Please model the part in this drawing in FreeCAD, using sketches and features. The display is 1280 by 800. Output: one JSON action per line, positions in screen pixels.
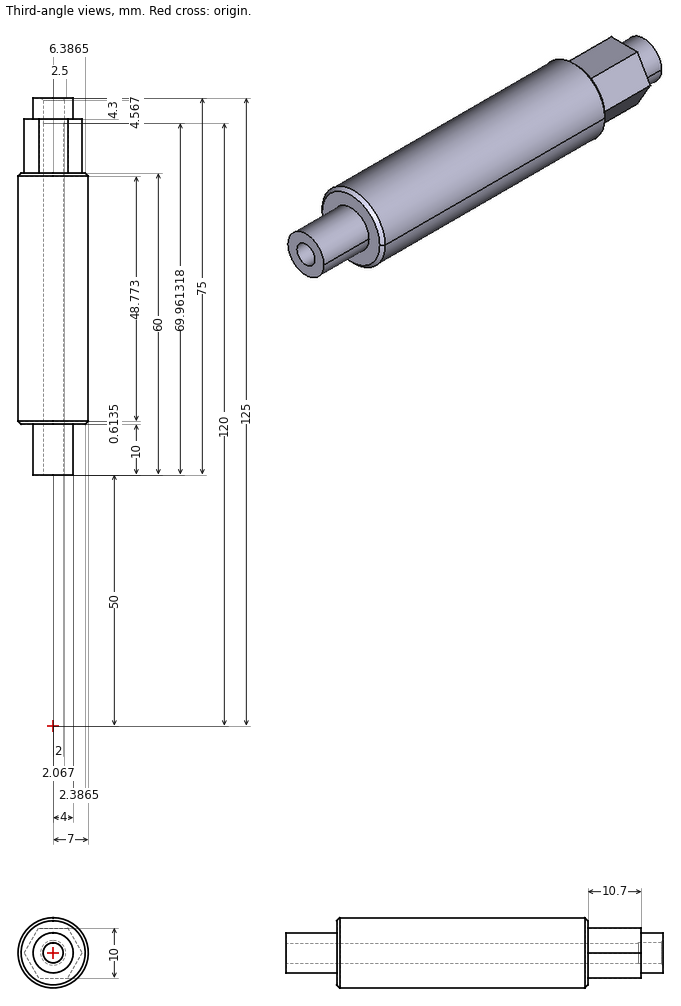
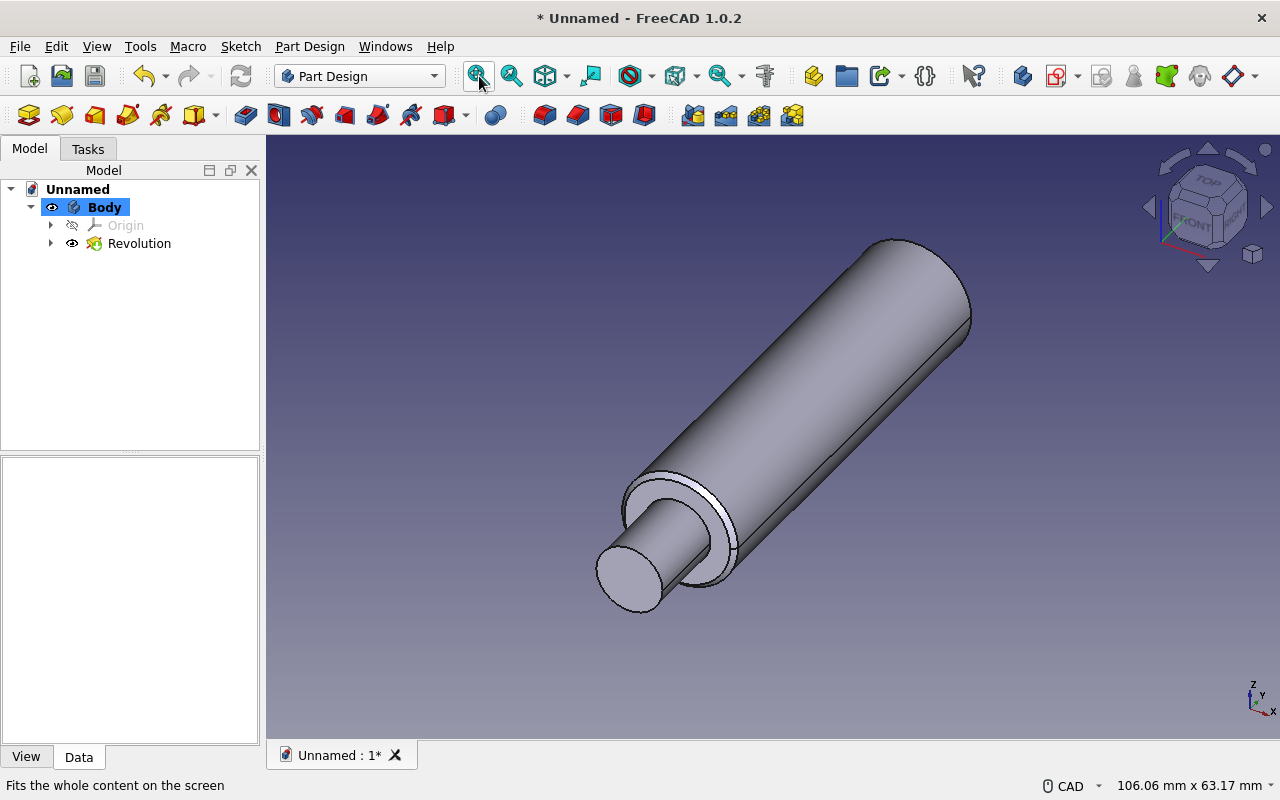
{"action": "key", "text": "4"}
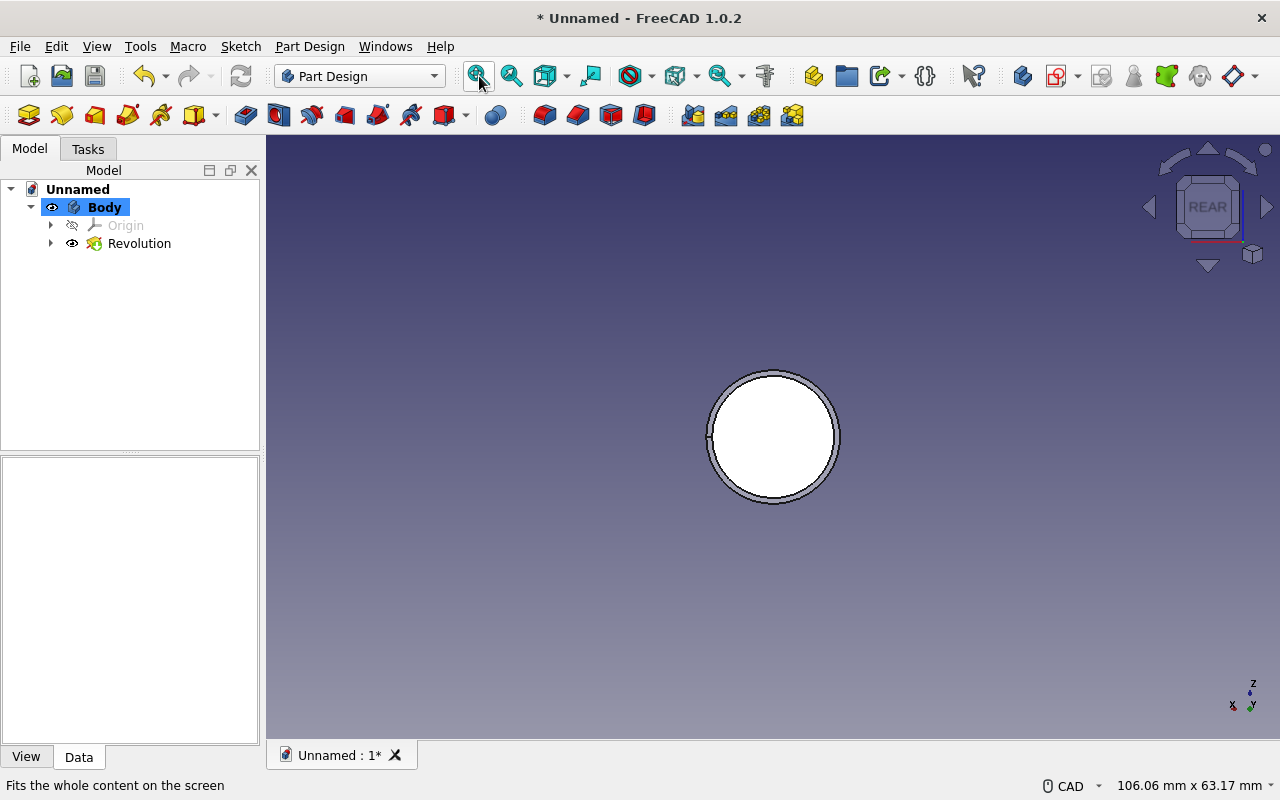
{"action": "left_click", "coordinate": [479, 76]}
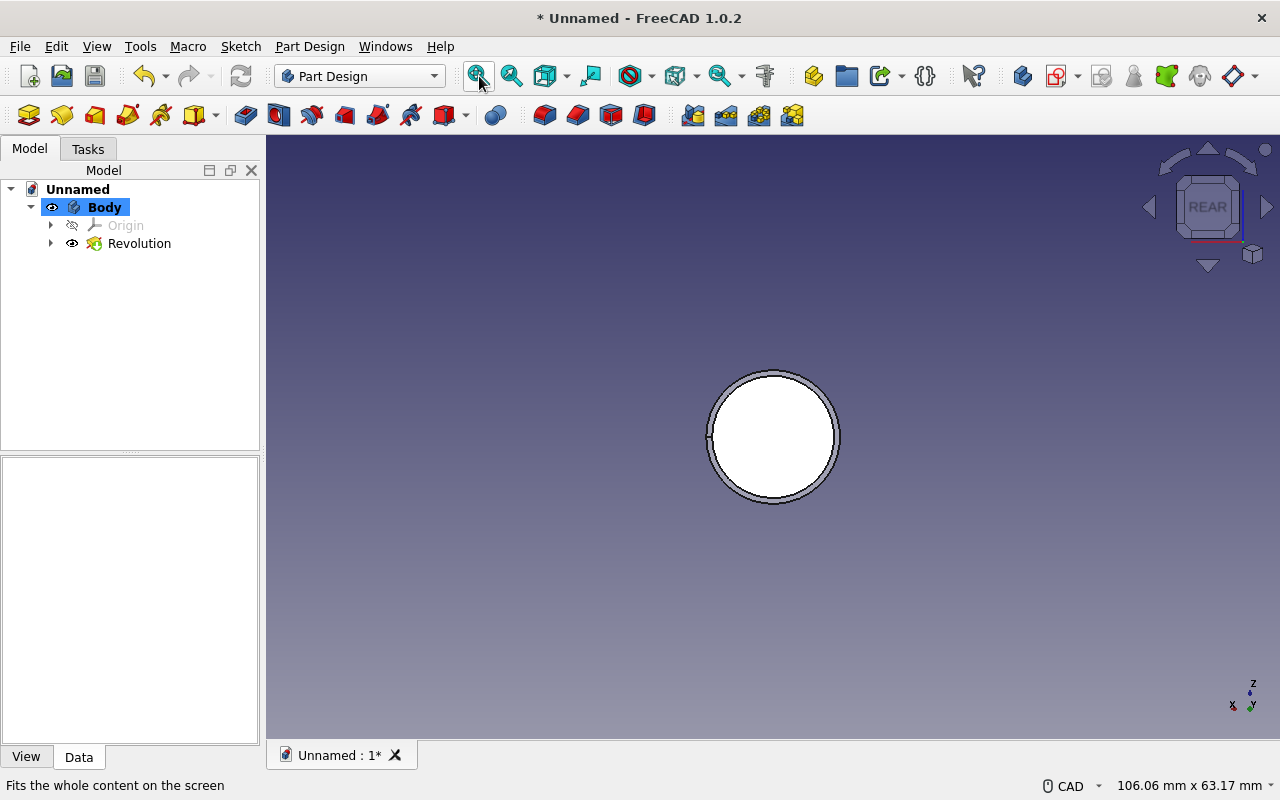
{"action": "left_click", "coordinate": [773, 436]}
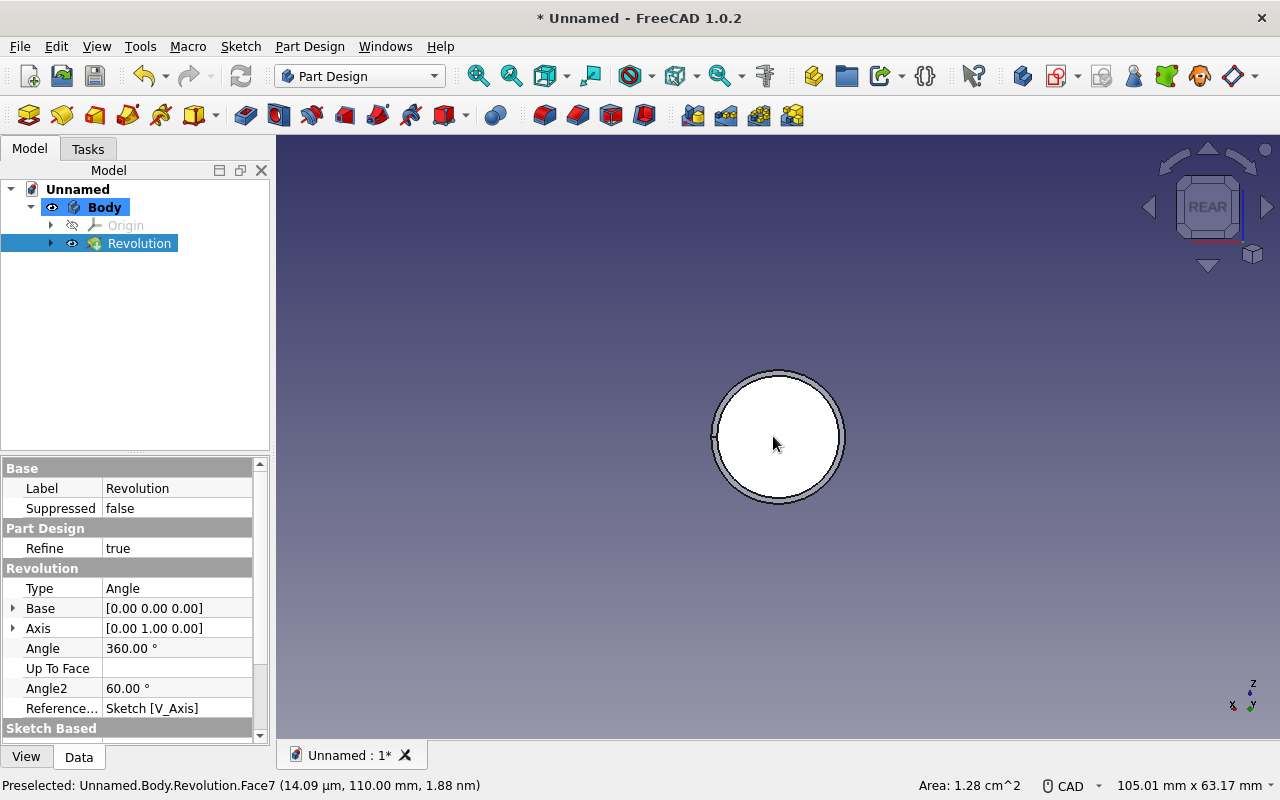
{"action": "left_click", "coordinate": [1056, 76]}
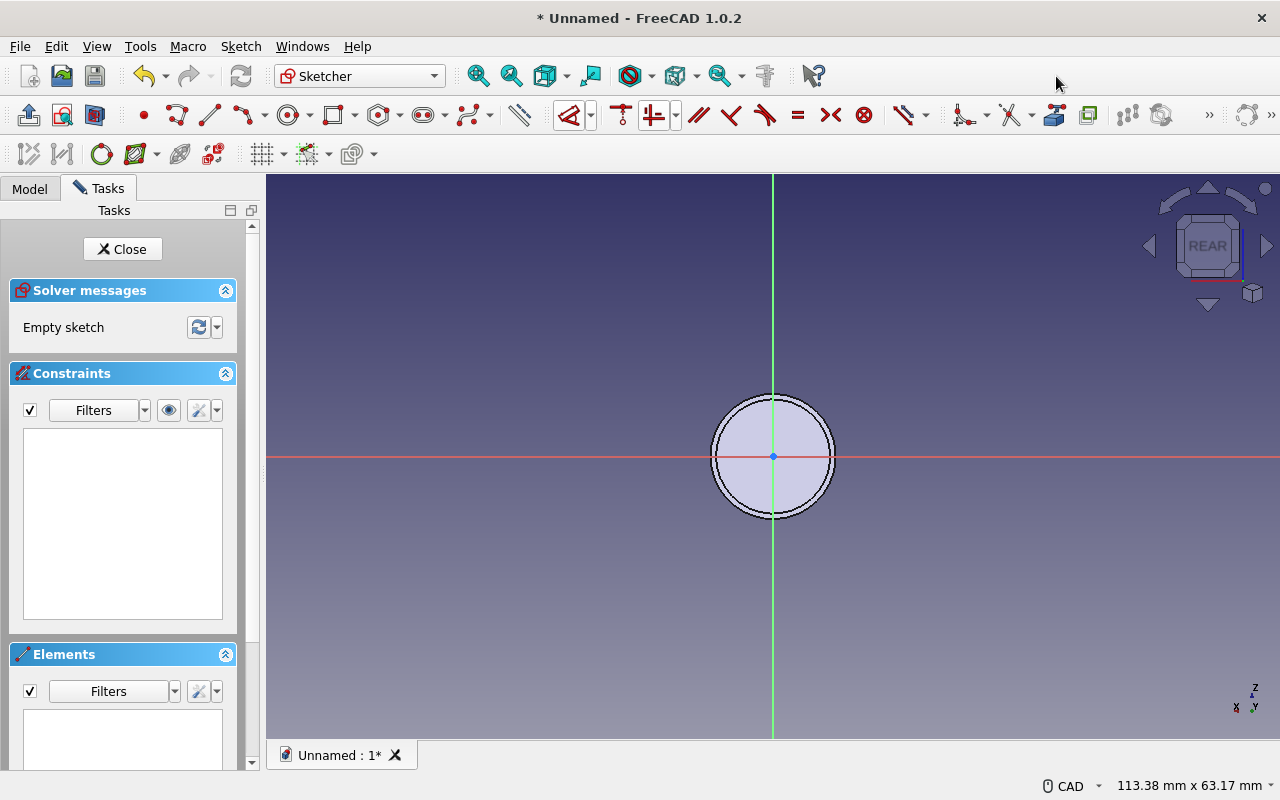
{"action": "scroll", "coordinate": [796, 456], "scroll_direction": "up", "scroll_amount": 7}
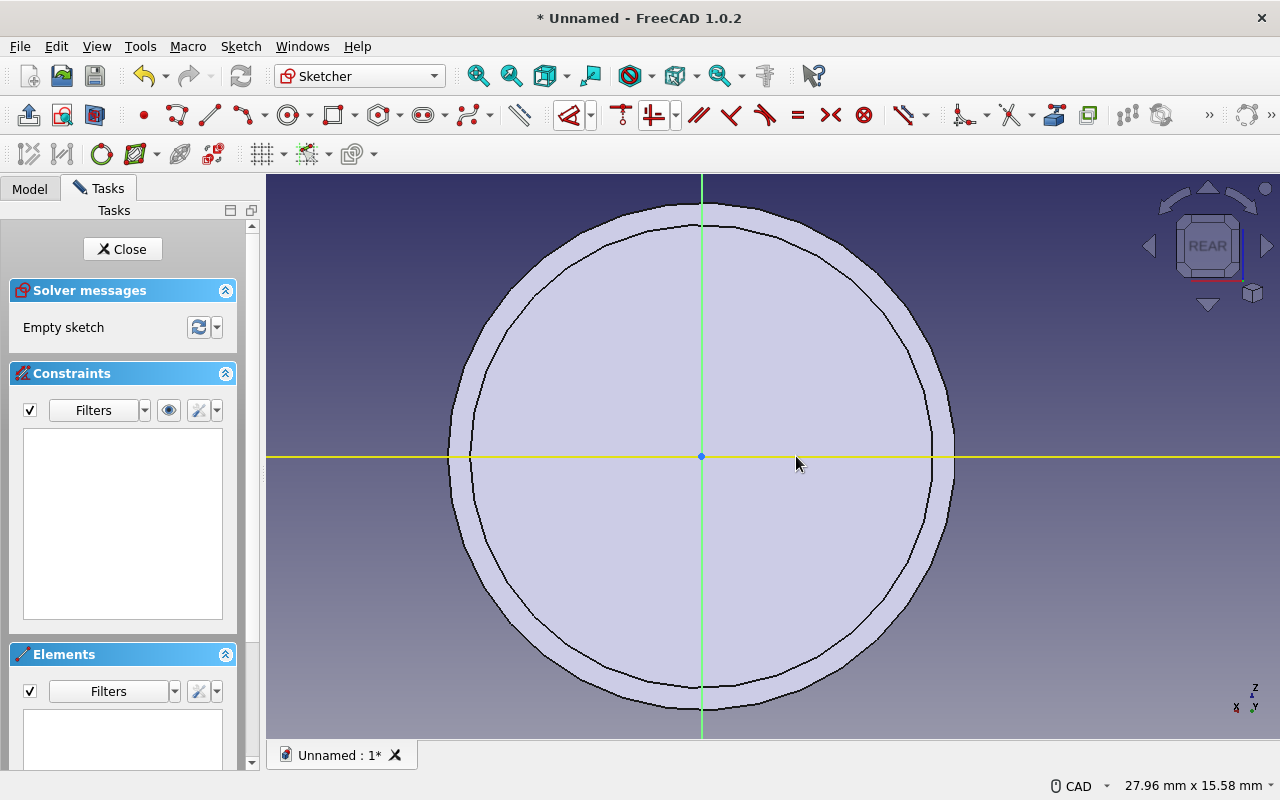
{"action": "left_click", "coordinate": [378, 116]}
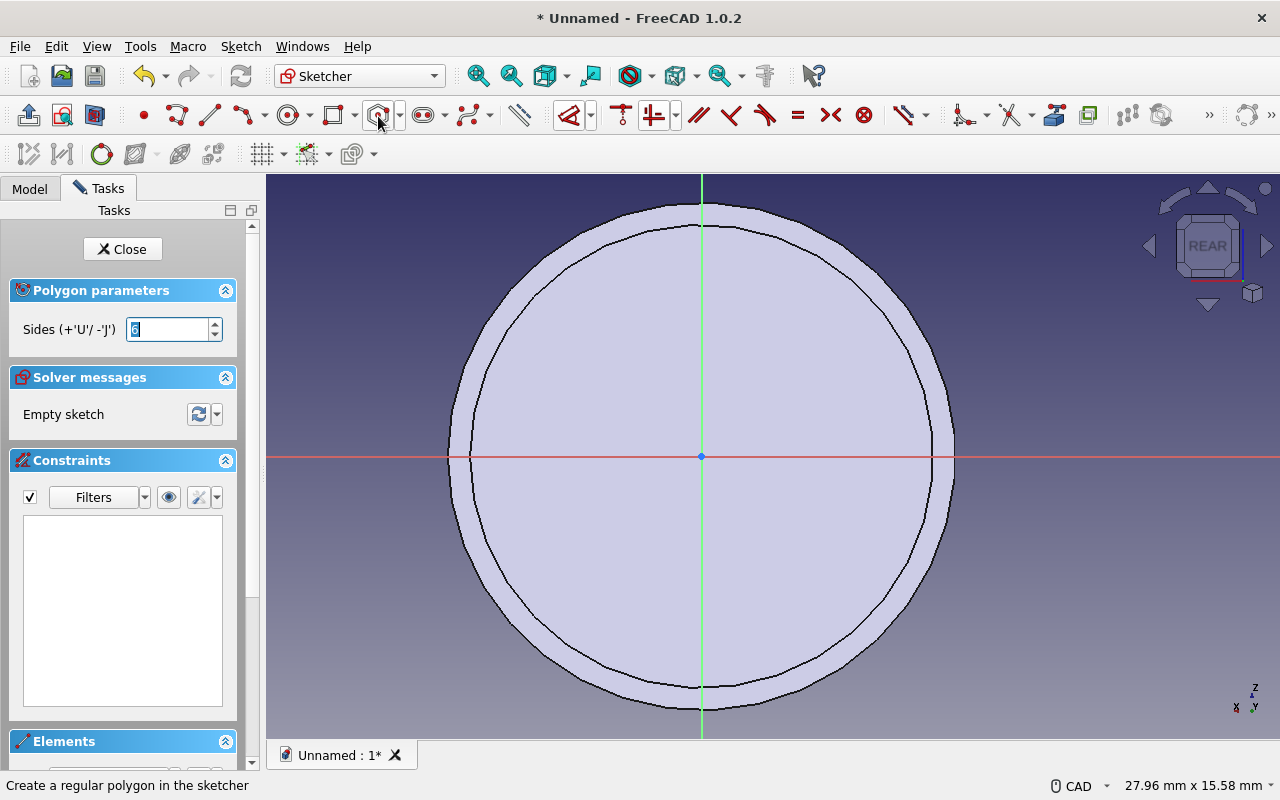
{"action": "left_click", "coordinate": [702, 456]}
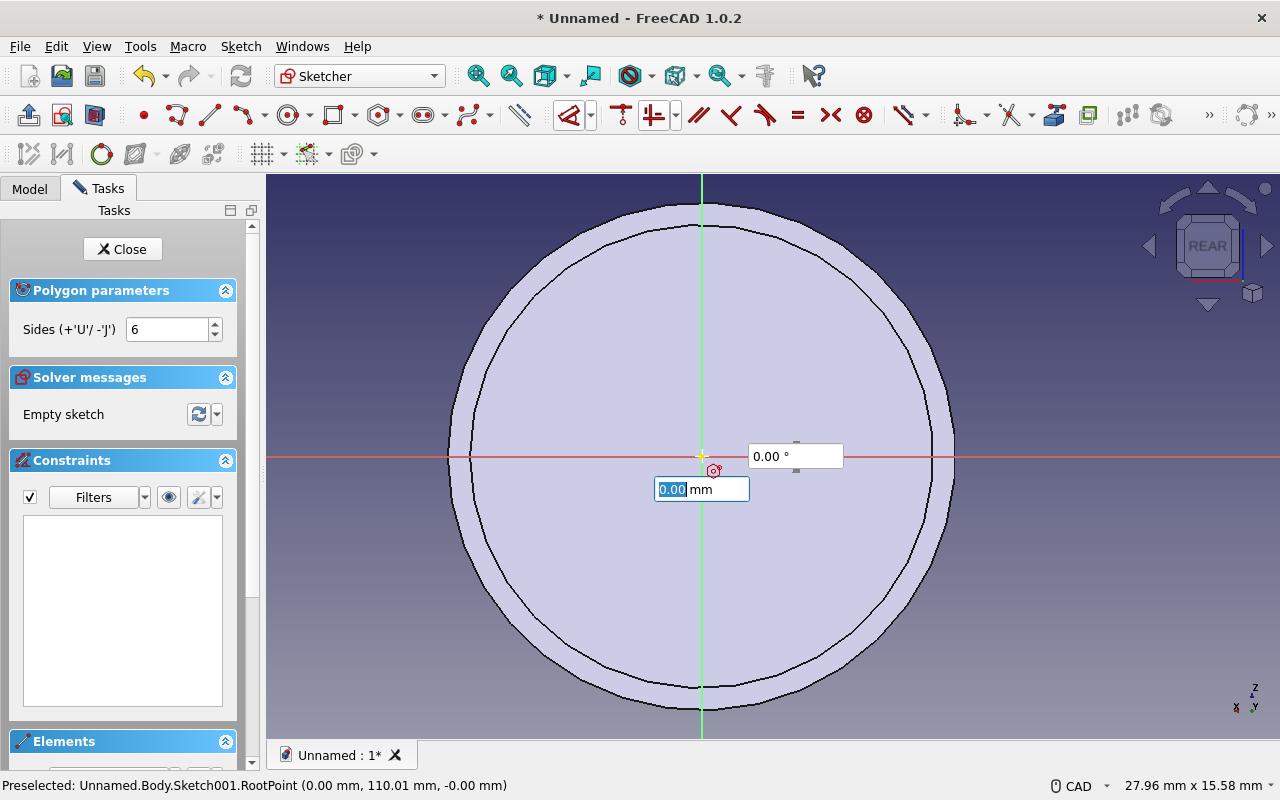
{"action": "left_click", "coordinate": [911, 456]}
{"action": "right_click", "coordinate": [911, 456]}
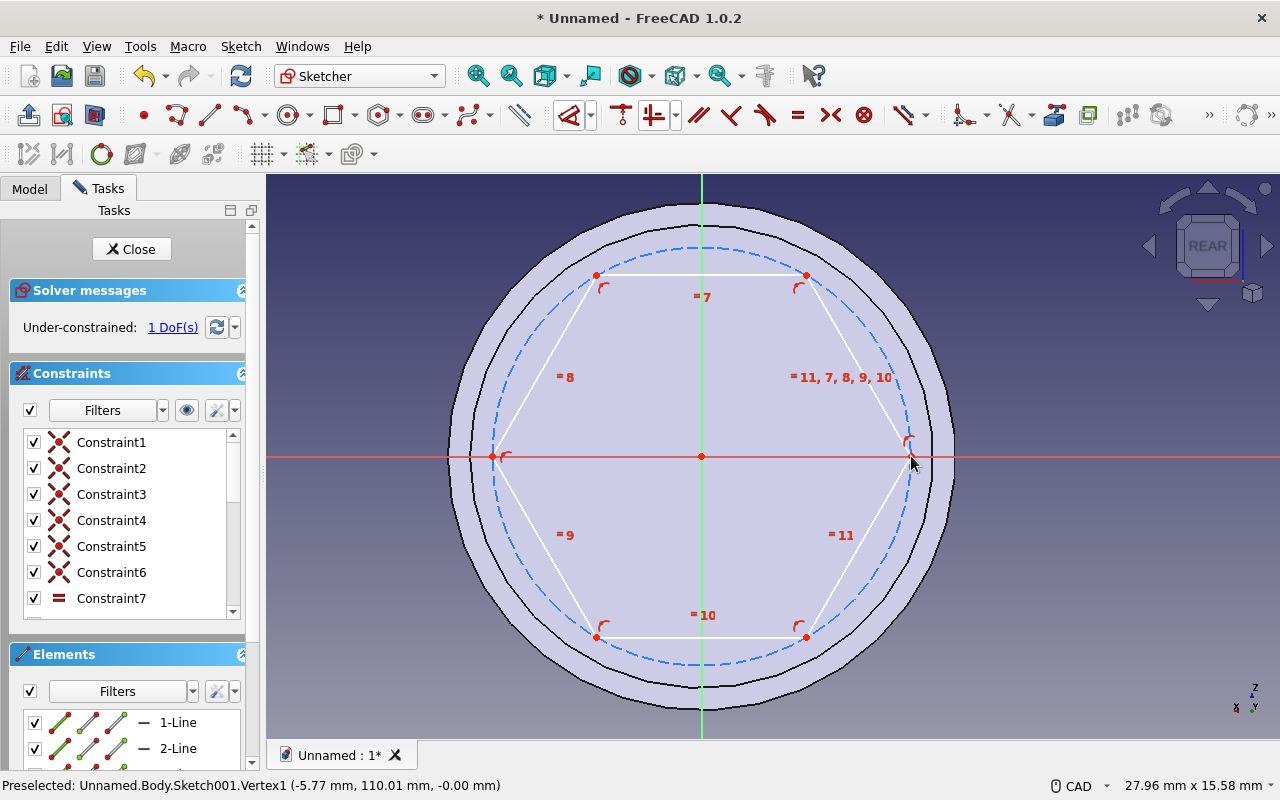
{"action": "left_click", "coordinate": [597, 638]}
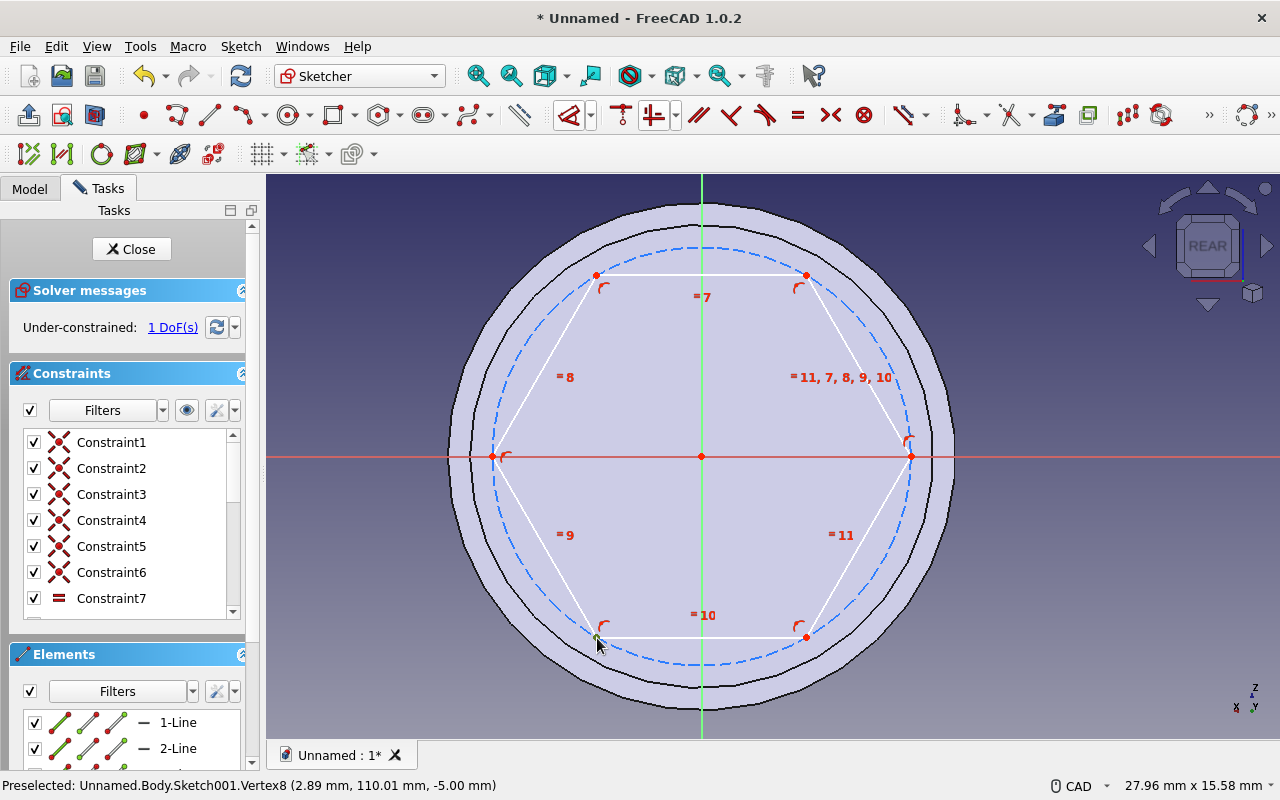
{"action": "left_click", "coordinate": [806, 275]}